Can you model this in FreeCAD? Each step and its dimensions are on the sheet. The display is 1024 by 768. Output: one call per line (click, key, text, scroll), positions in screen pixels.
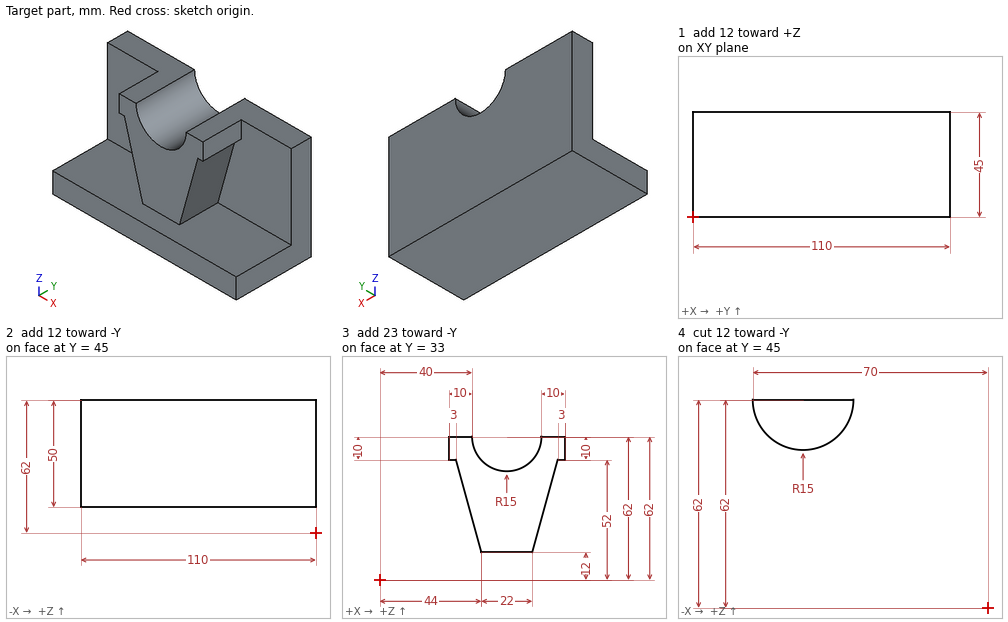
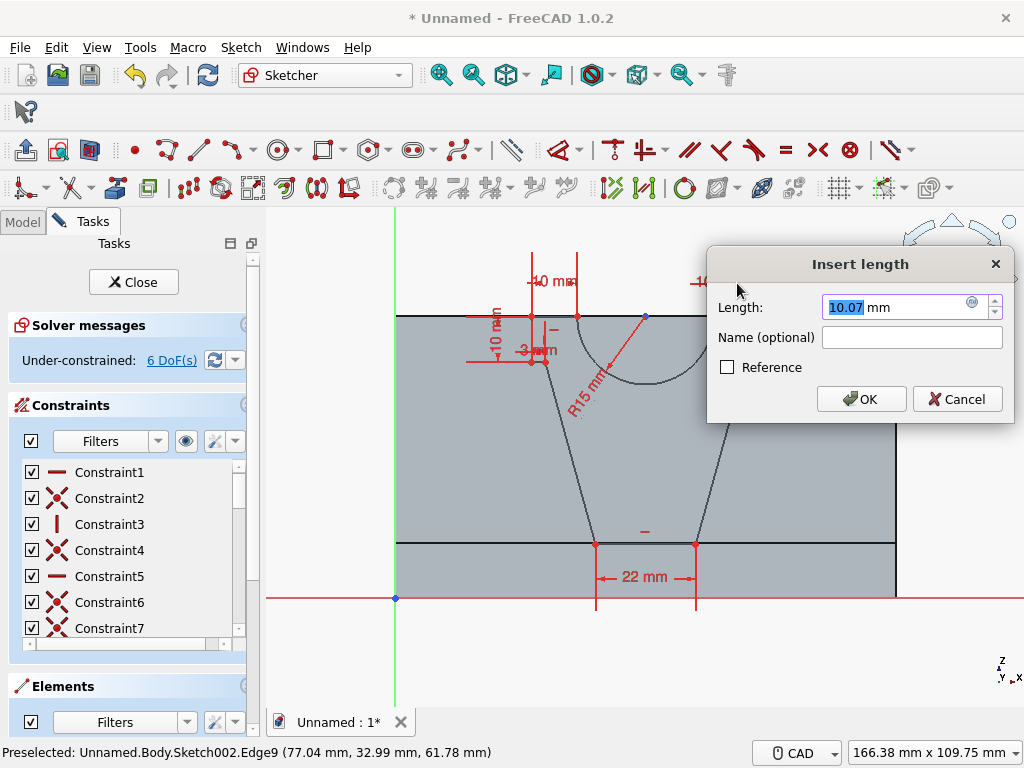
text(10)
key(Return)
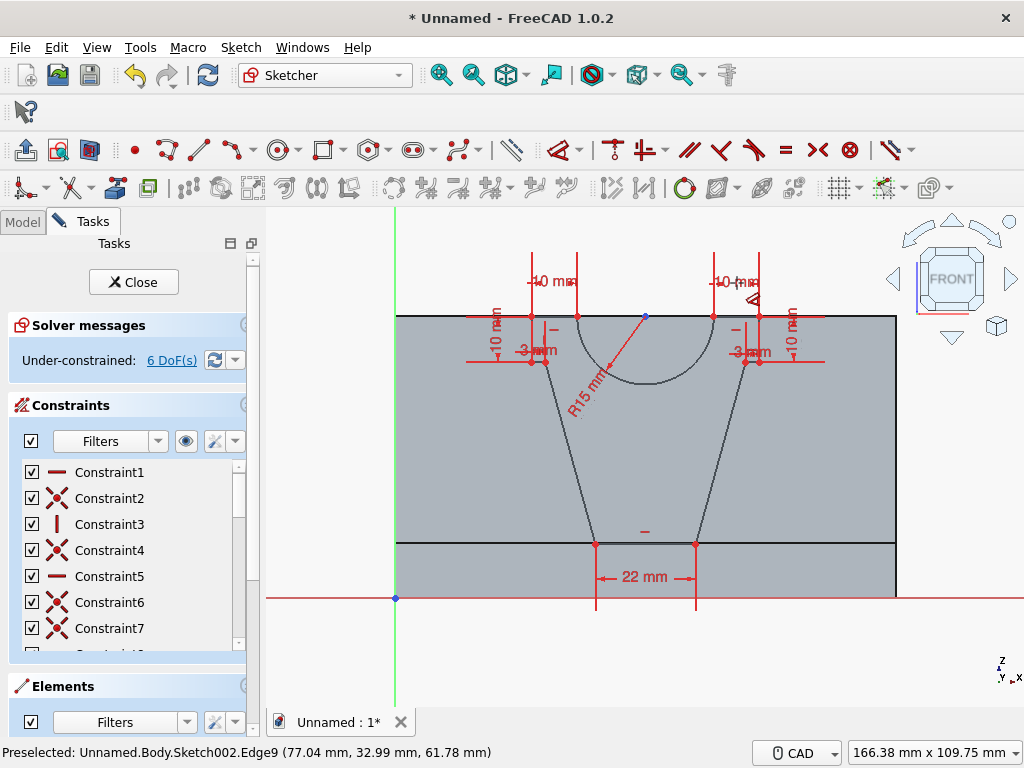
click(577, 317)
click(486, 632)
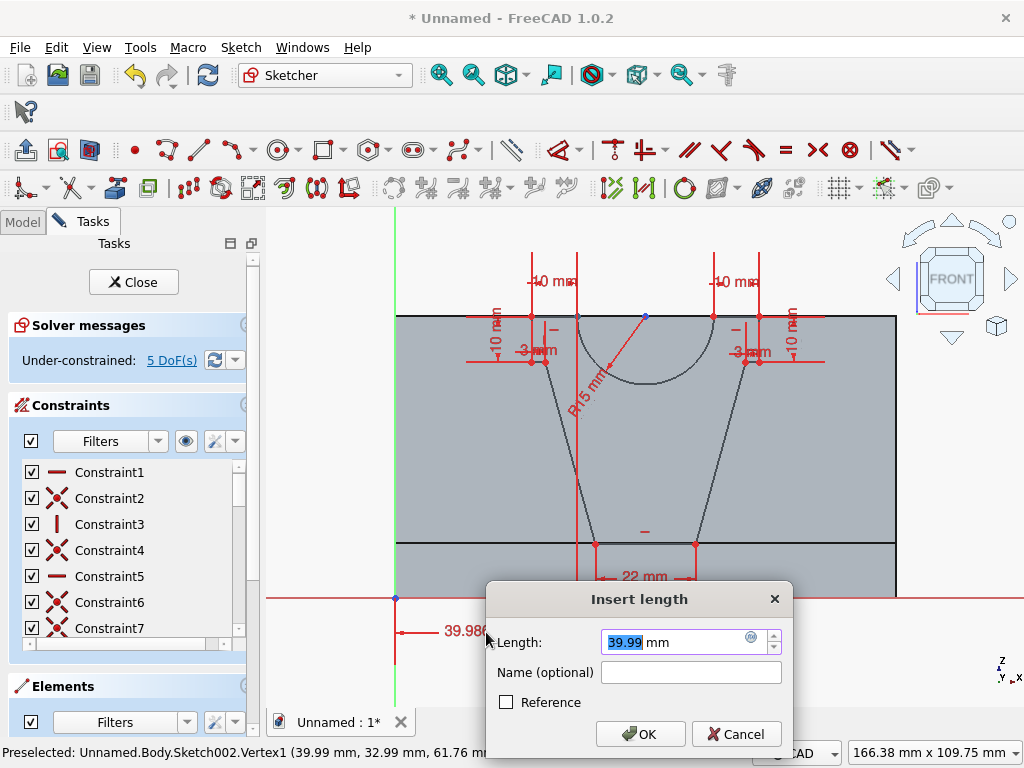
text(40)
key(Return)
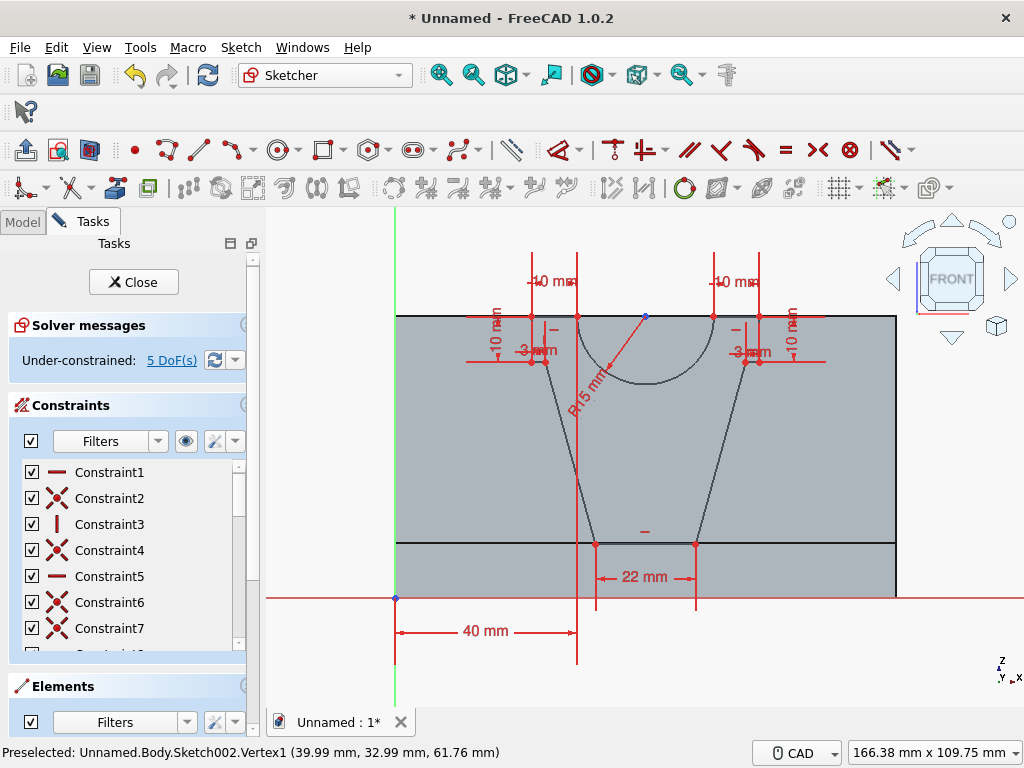
click(577, 317)
click(361, 457)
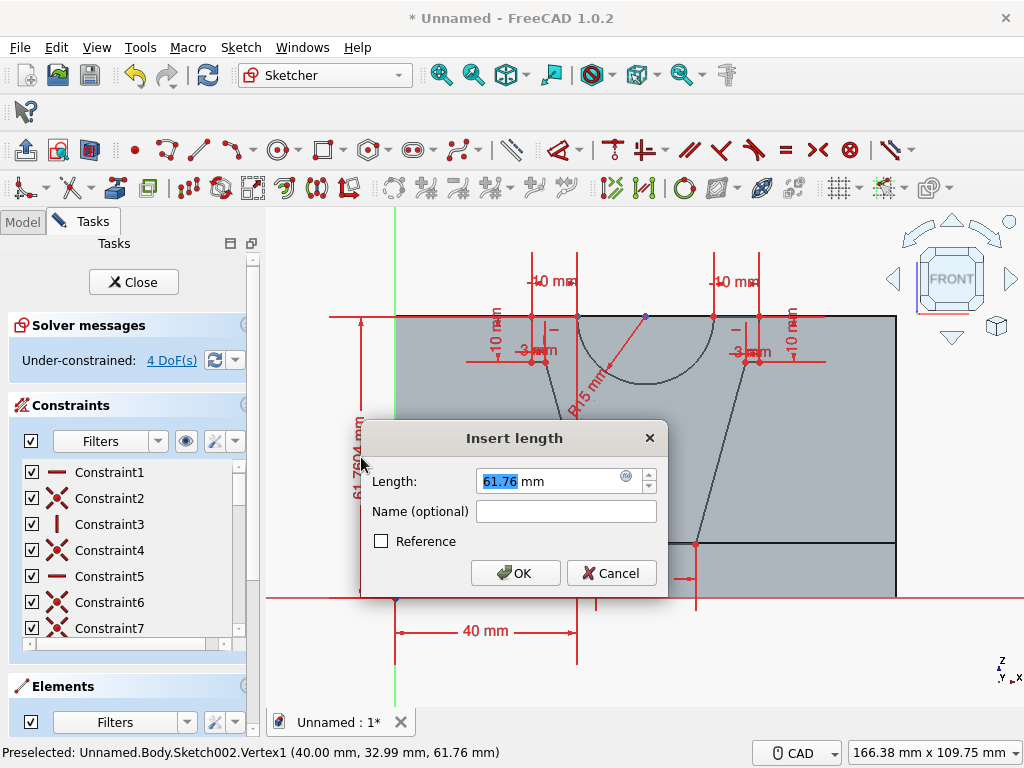
text(62)
key(Return)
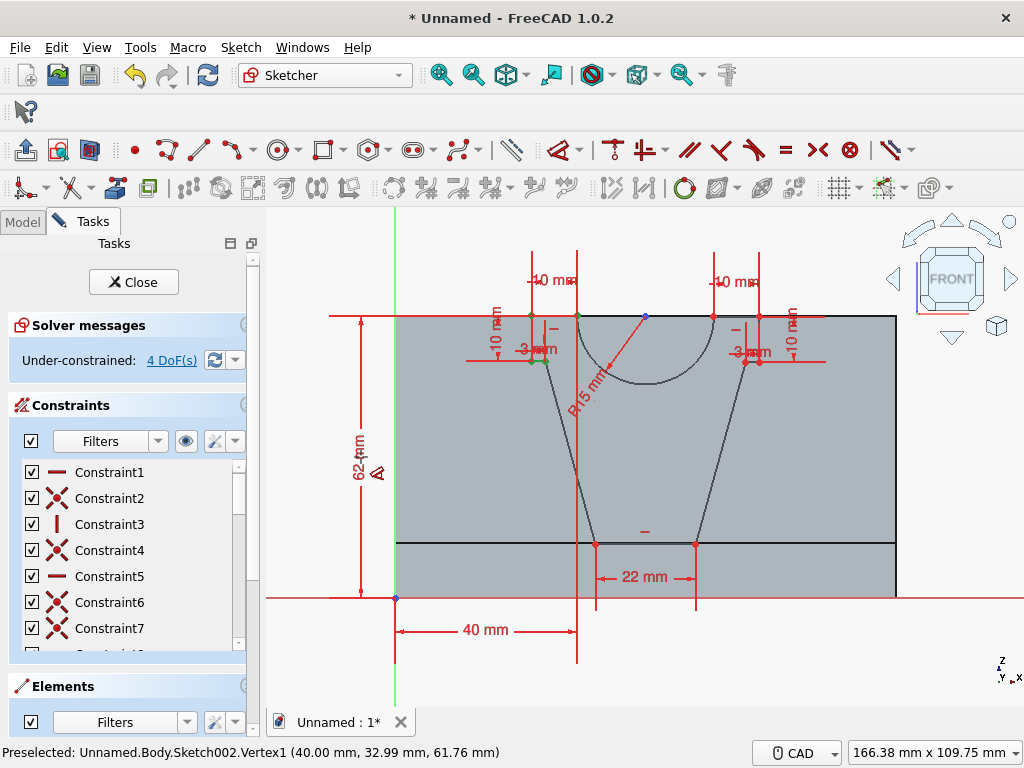
click(596, 544)
click(565, 632)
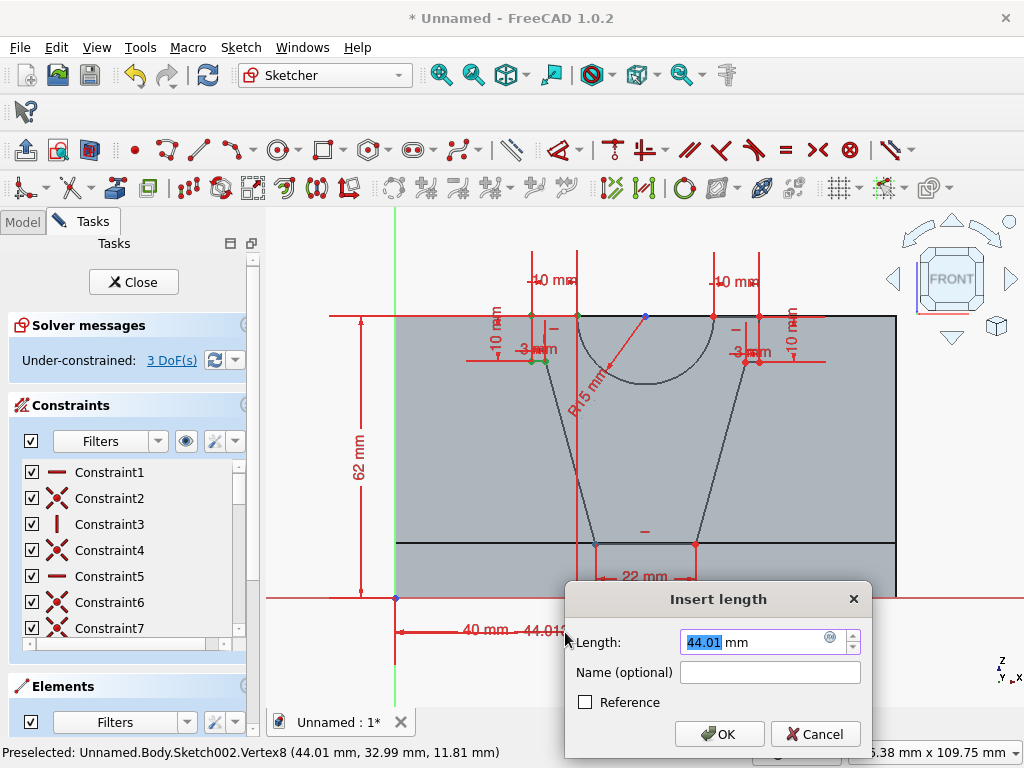
text(44)
key(Return)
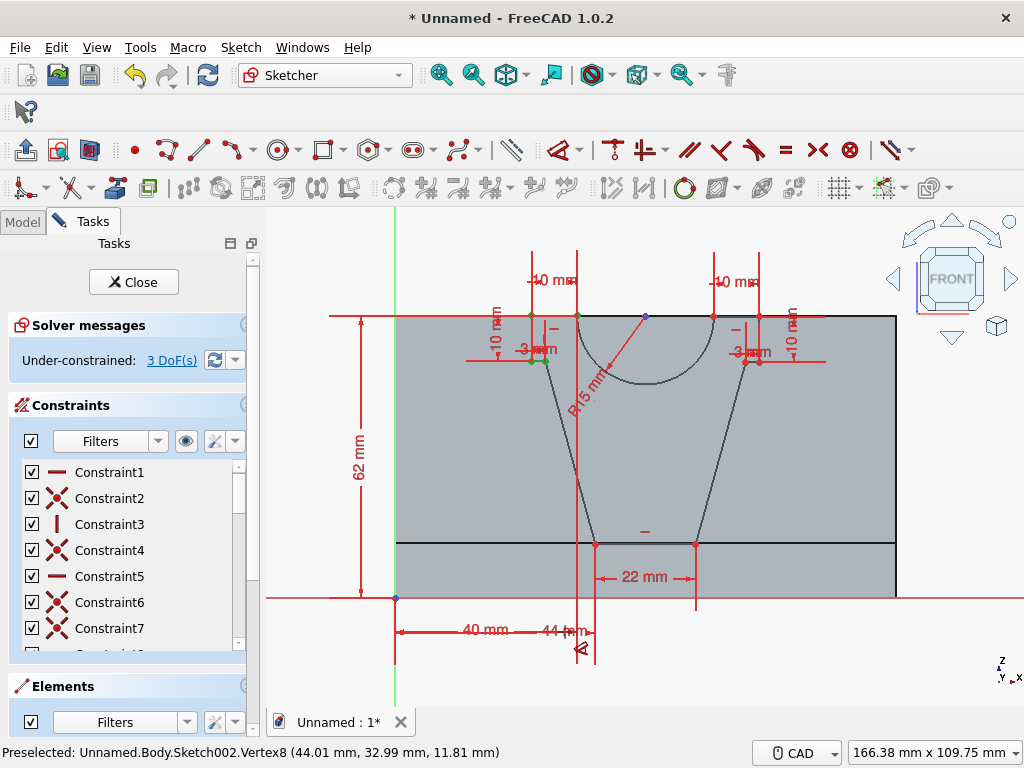
click(595, 544)
click(361, 571)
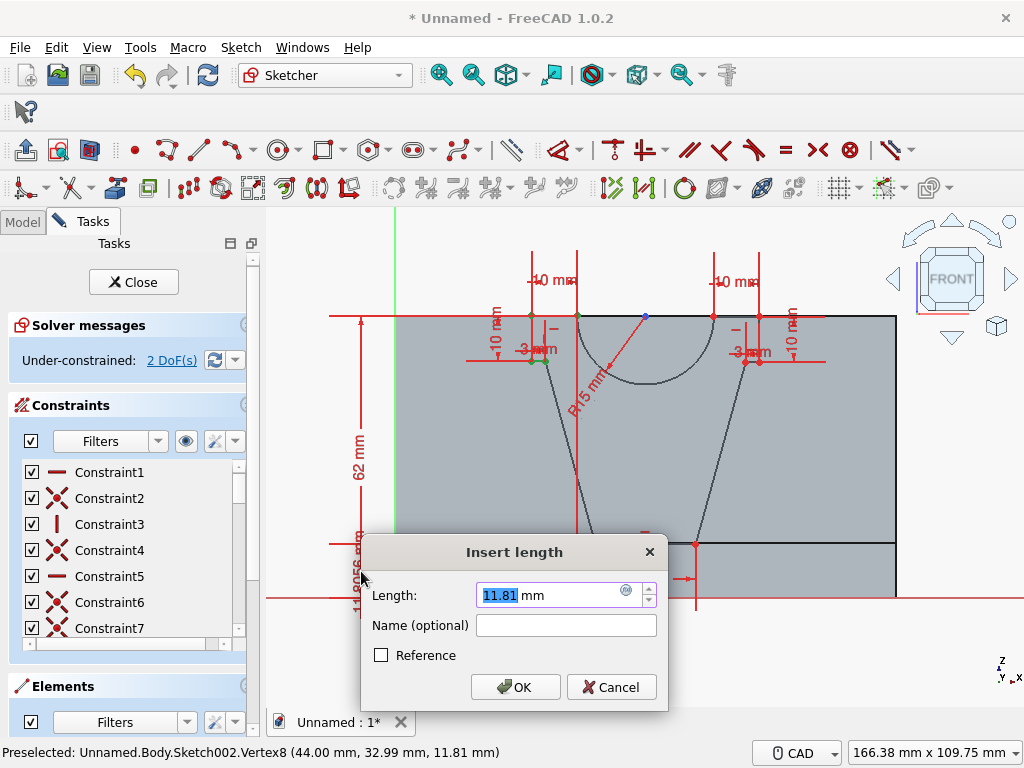
text(12)
key(Return)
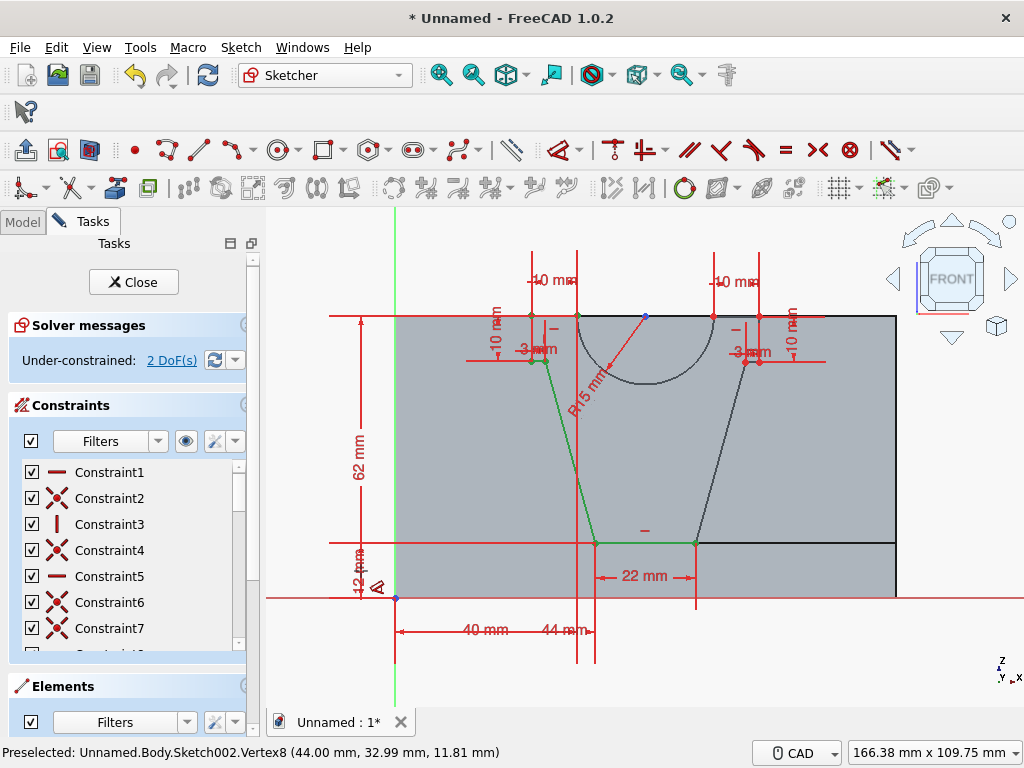
click(746, 362)
click(361, 480)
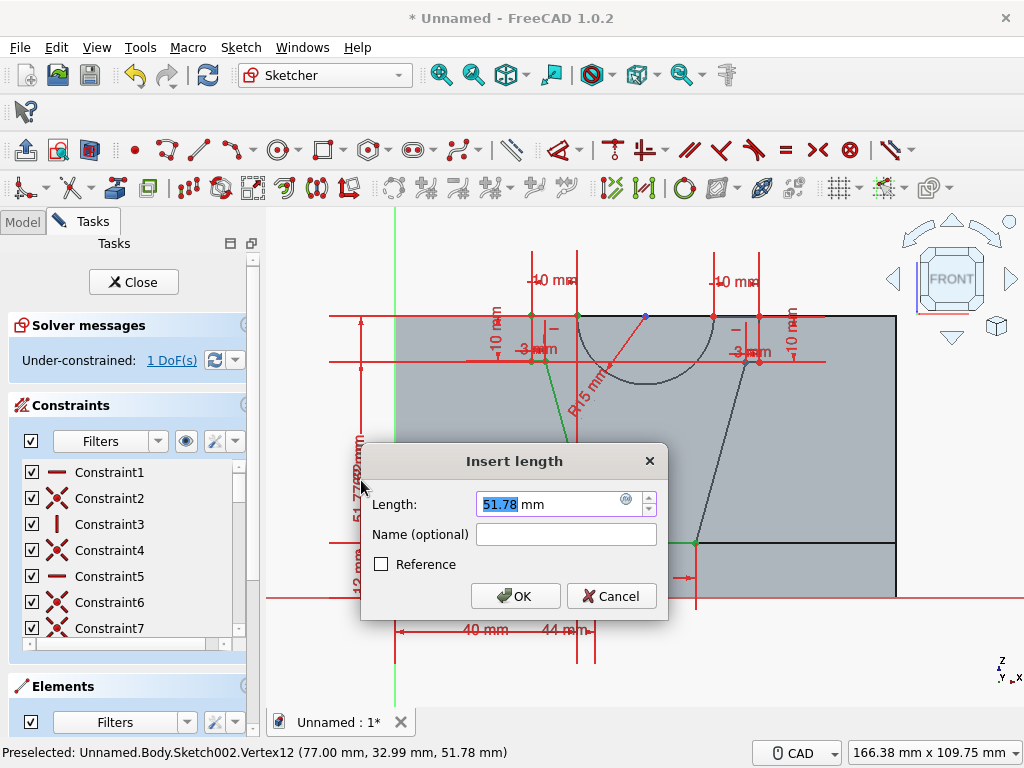
text(52)
key(Return)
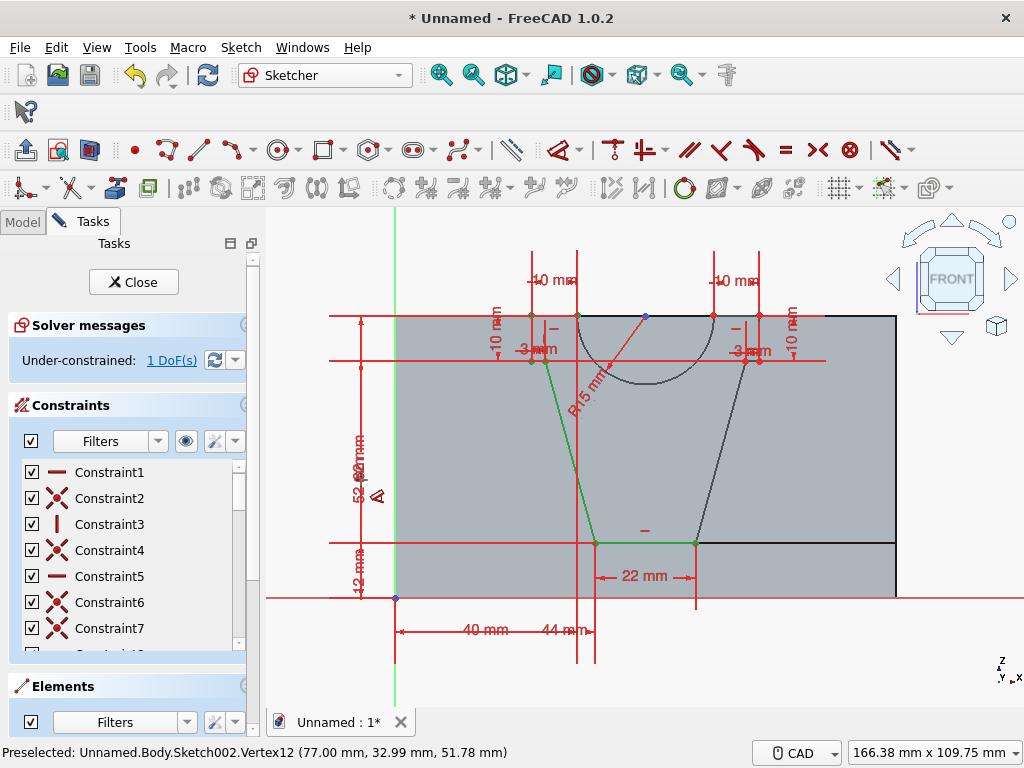
click(646, 316)
click(361, 392)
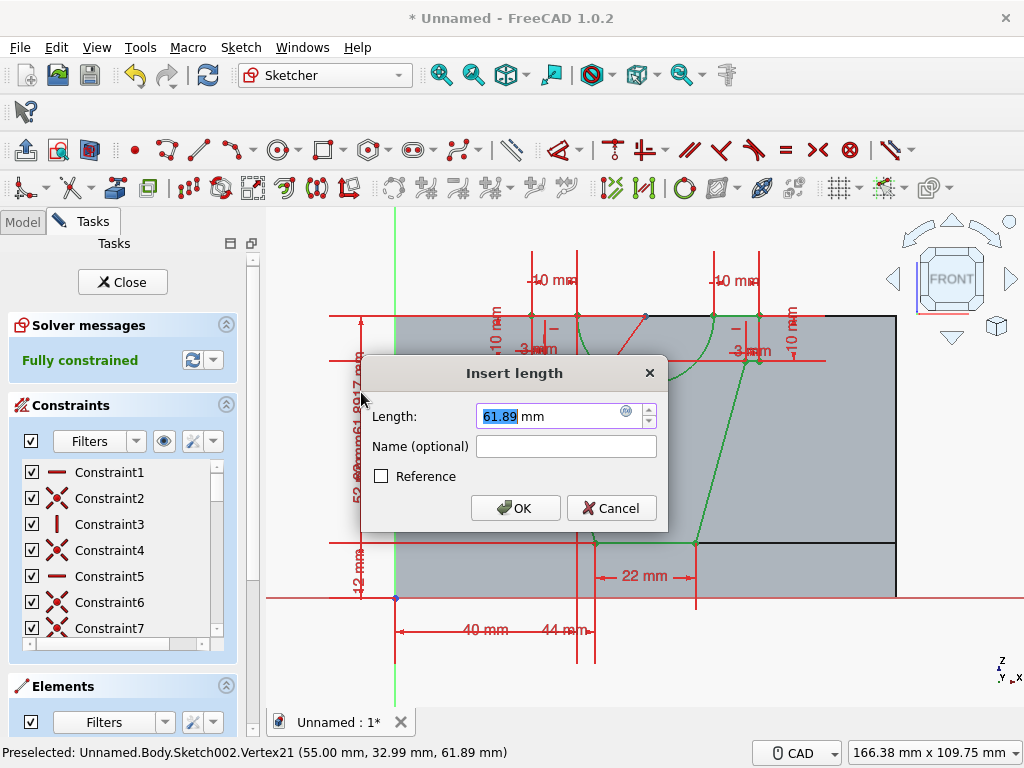
text(62)
key(Return)
key(Escape)